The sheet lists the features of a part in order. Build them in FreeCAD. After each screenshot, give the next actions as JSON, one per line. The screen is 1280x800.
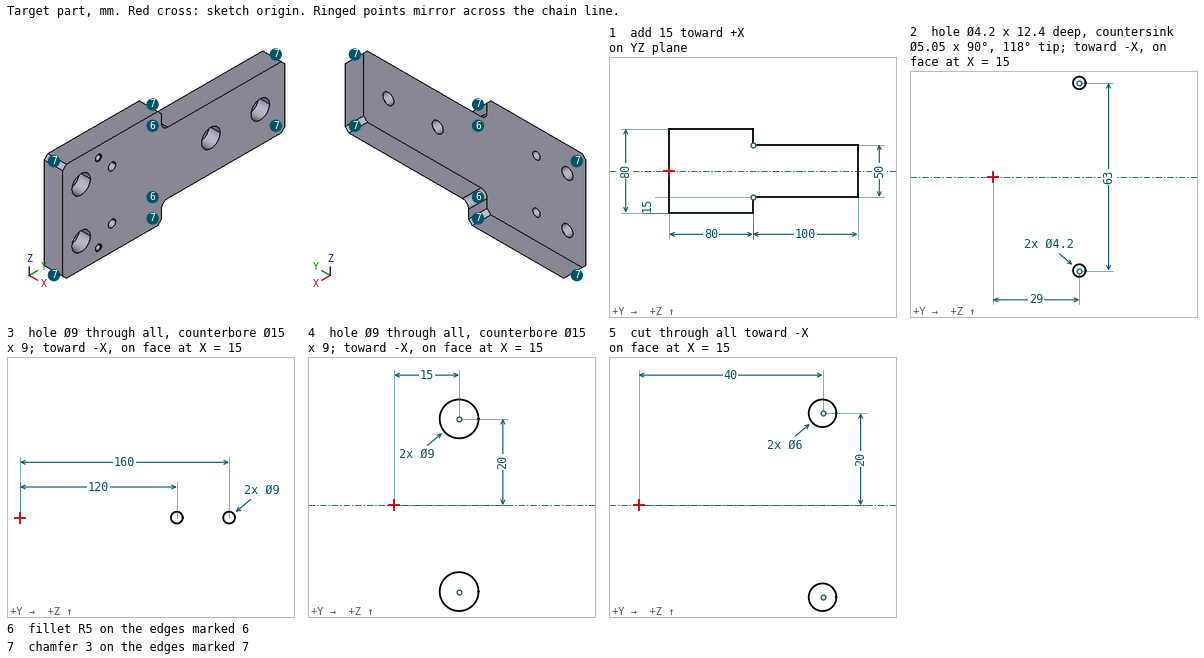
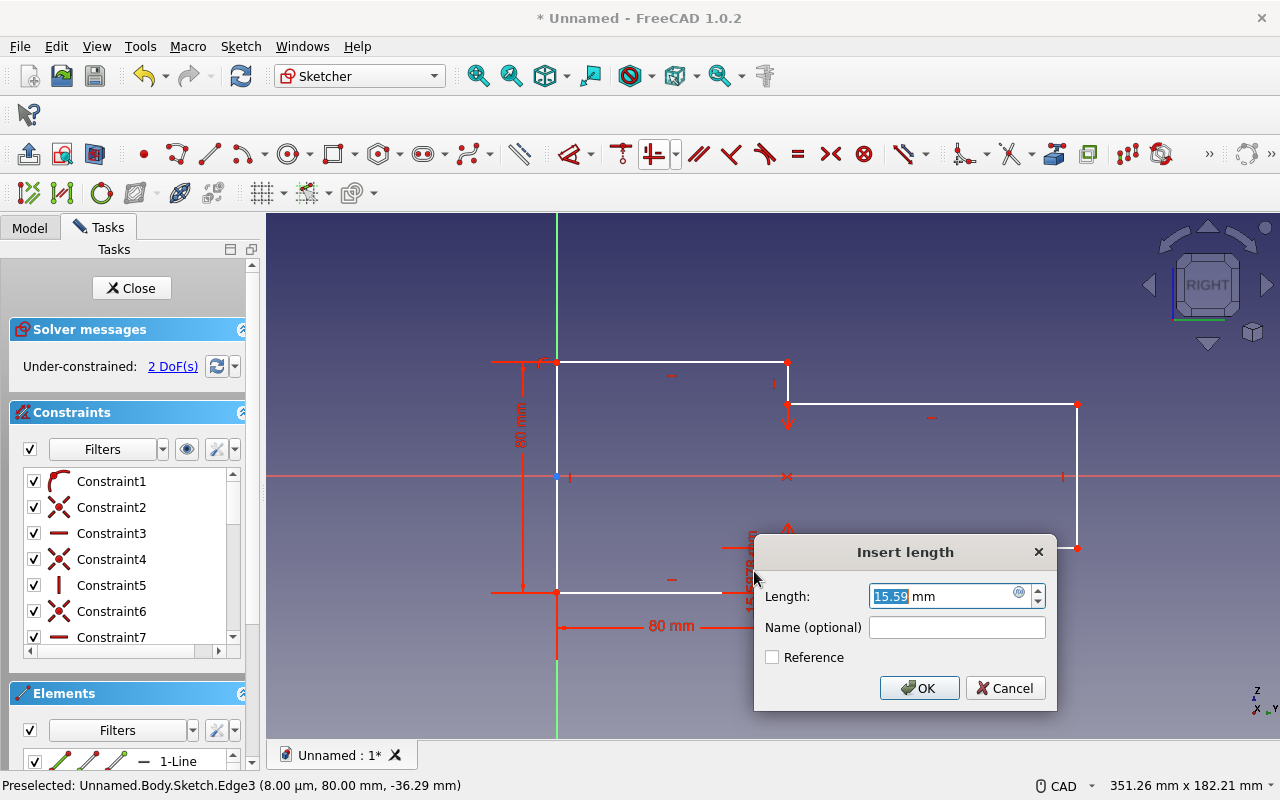
{"action": "type", "text": "15"}
{"action": "key", "text": "Return"}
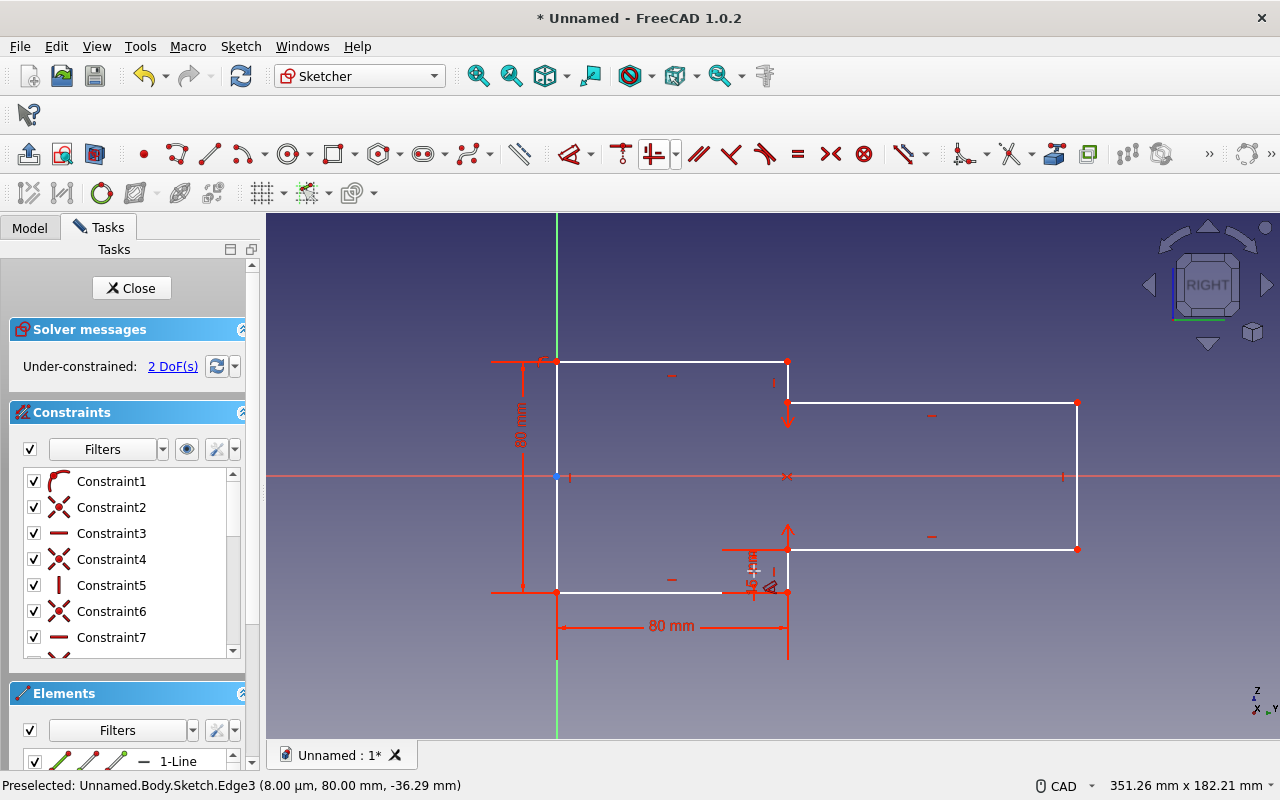
{"action": "left_click", "coordinate": [1077, 506]}
{"action": "left_click", "coordinate": [1111, 442]}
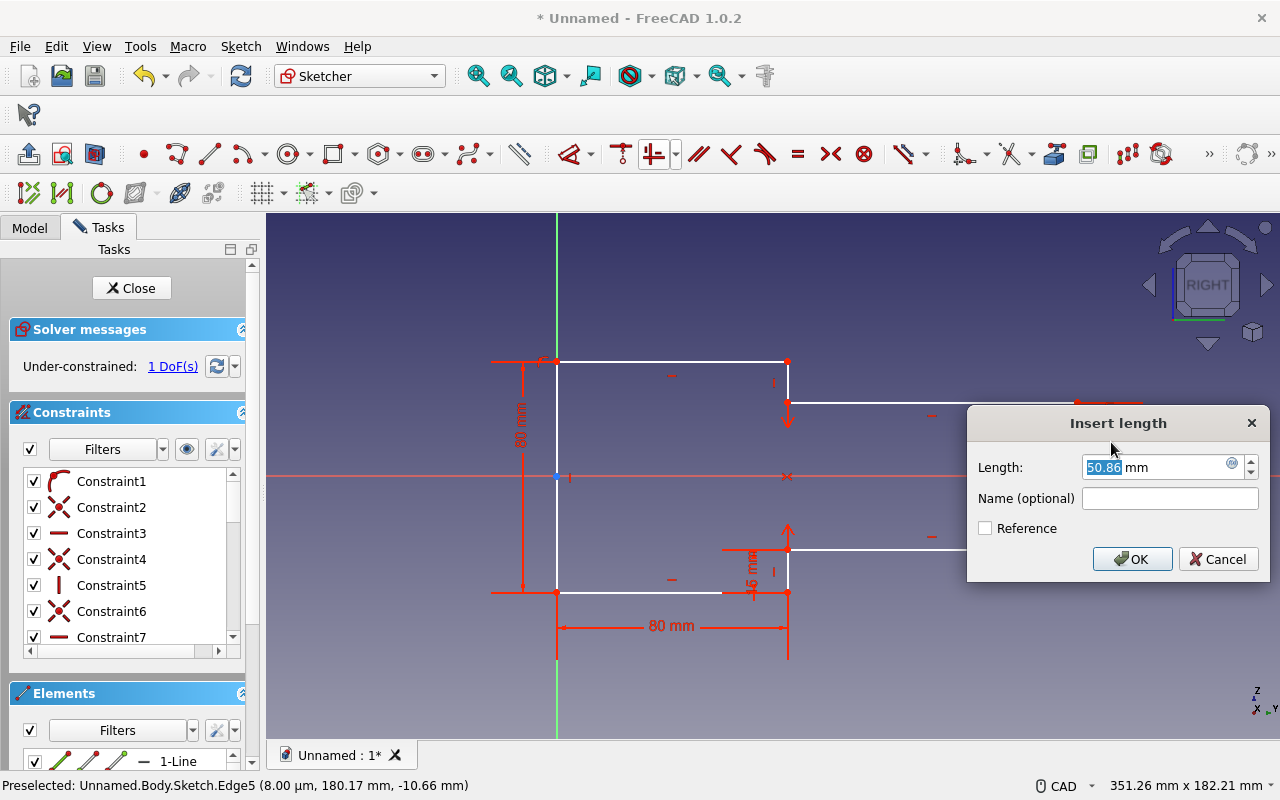
{"action": "type", "text": "50"}
{"action": "key", "text": "Return"}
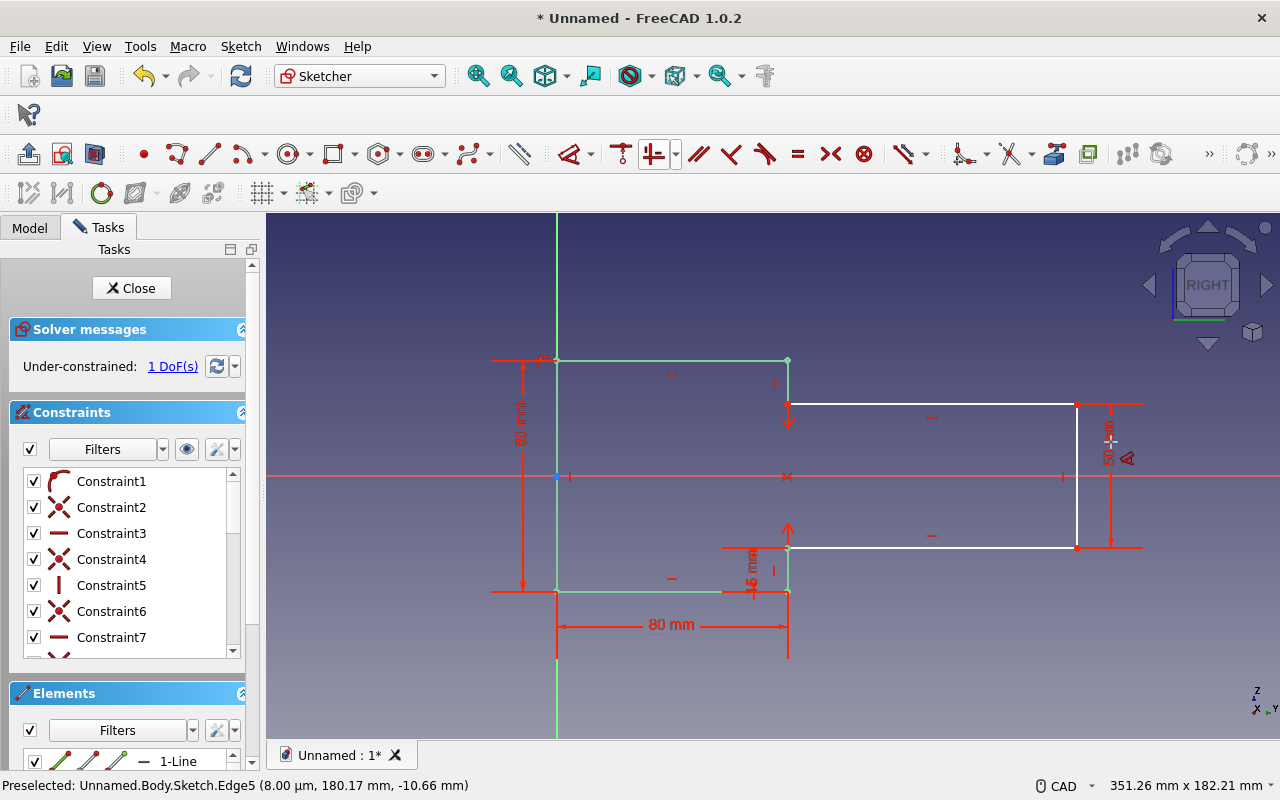
{"action": "left_click", "coordinate": [875, 548]}
{"action": "left_click", "coordinate": [932, 582]}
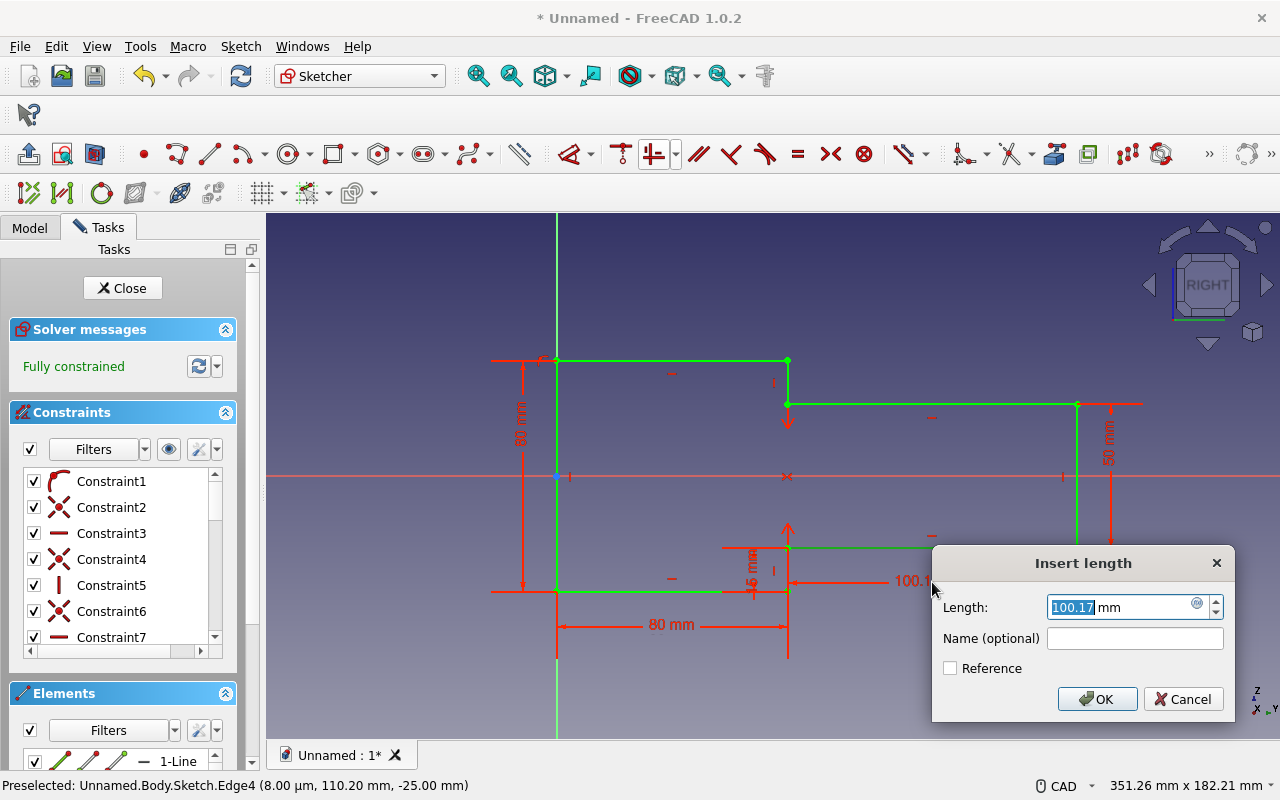
{"action": "type", "text": "100"}
{"action": "key", "text": "Return"}
{"action": "key", "text": "Escape"}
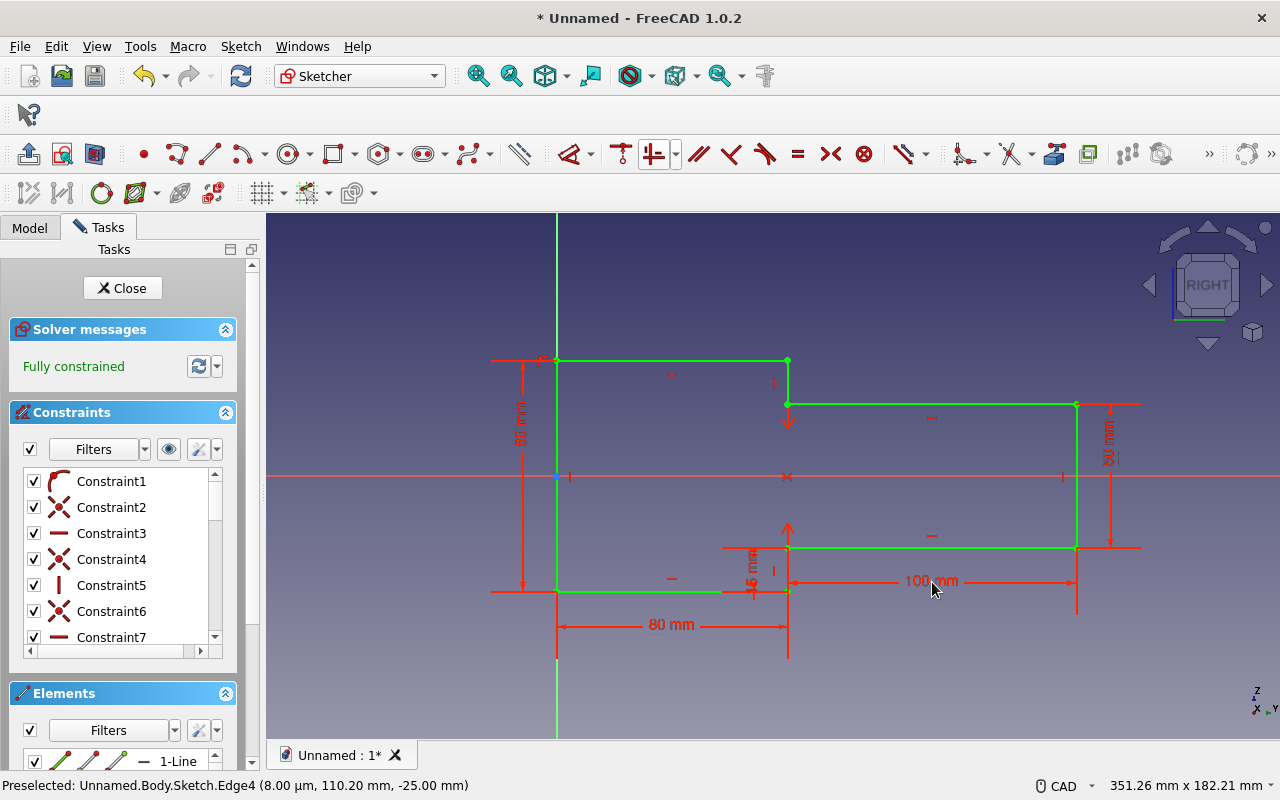
{"action": "left_click", "coordinate": [123, 288]}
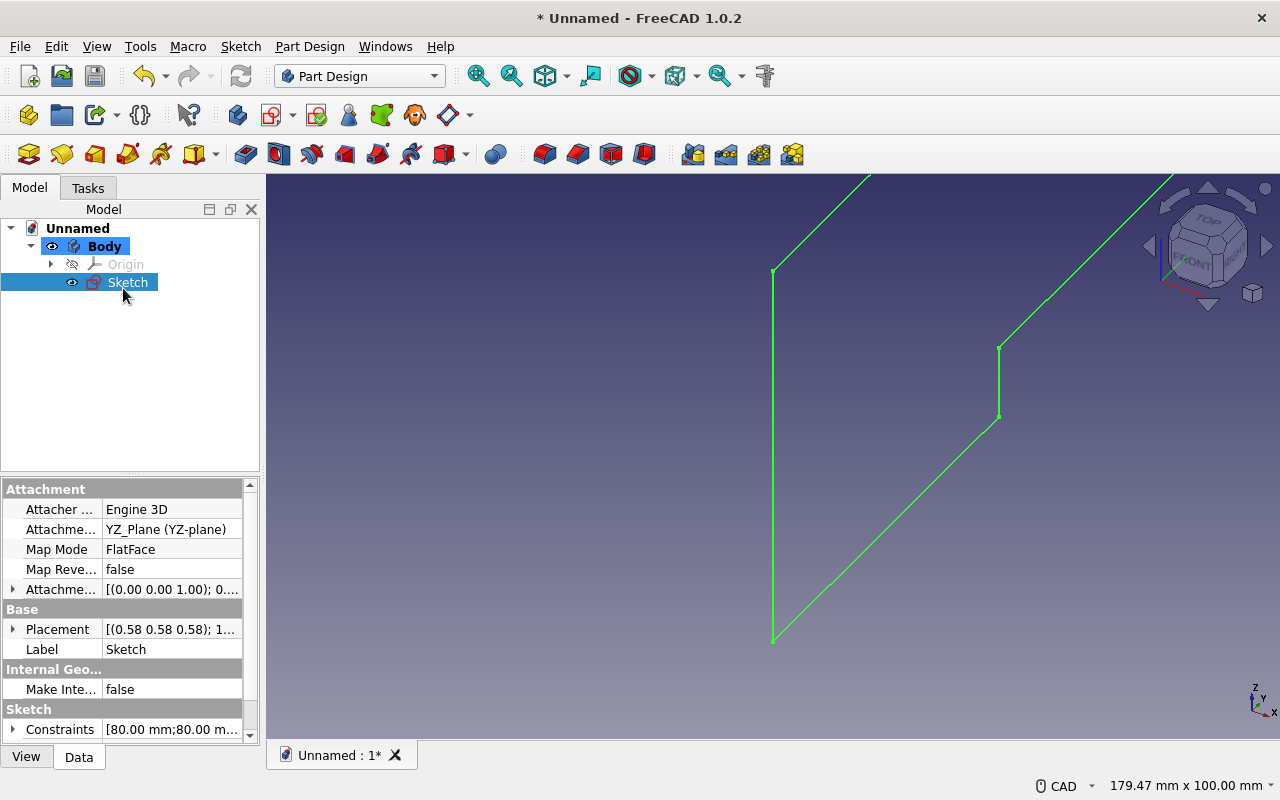
{"action": "left_click", "coordinate": [29, 154]}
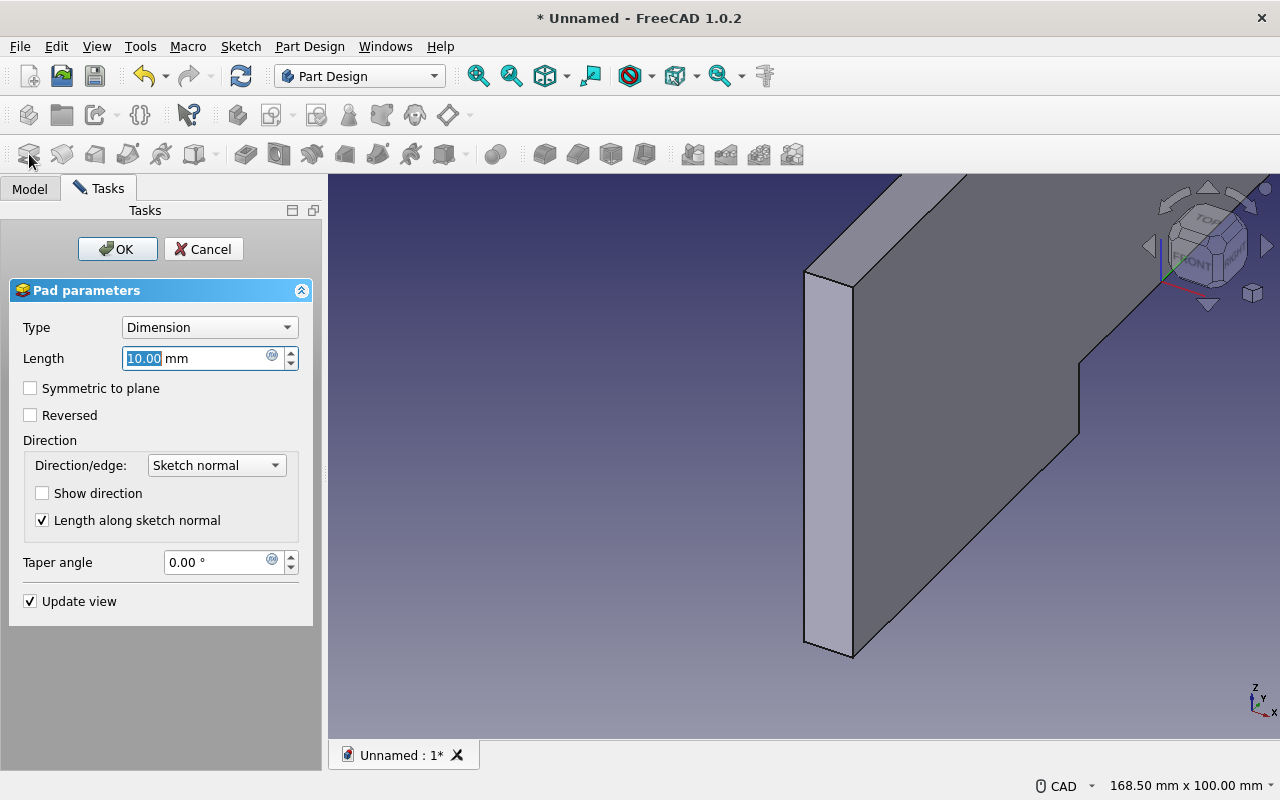
{"action": "type", "text": "15"}
{"action": "key", "text": "Tab"}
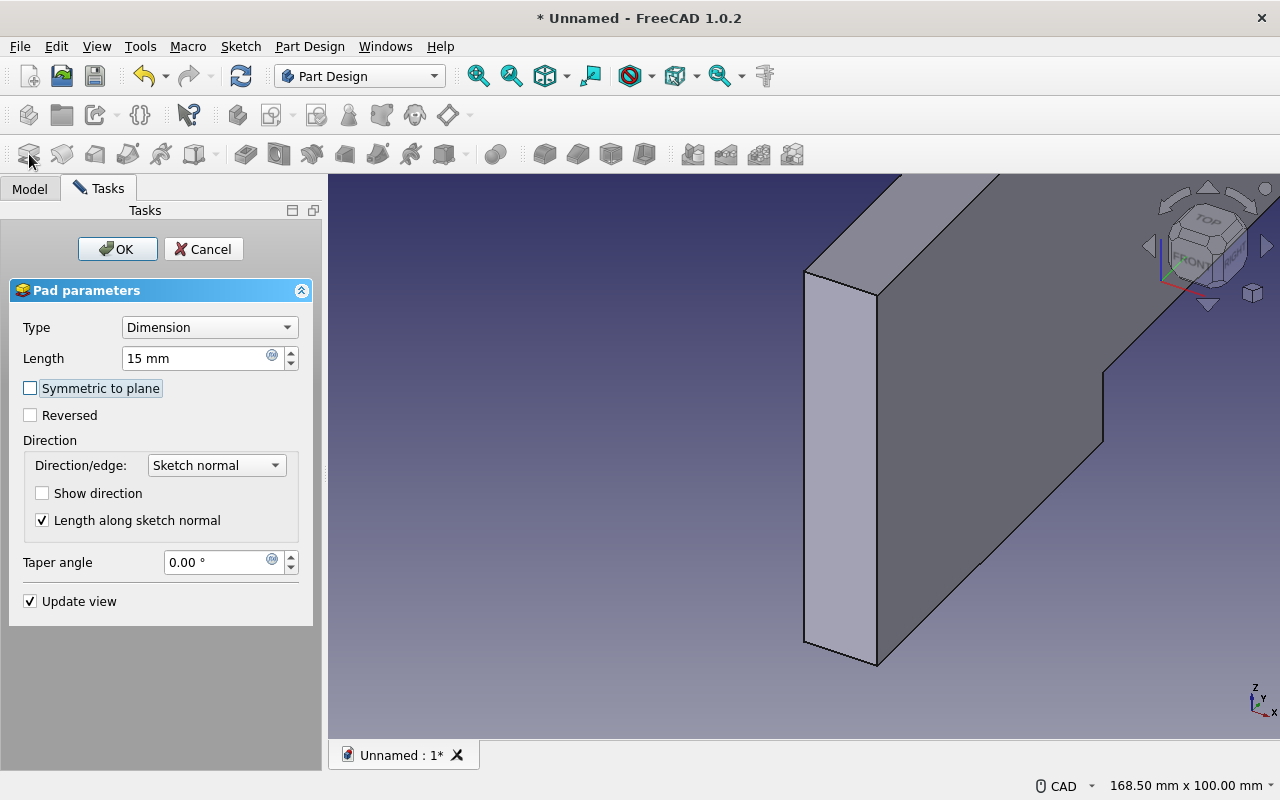
{"action": "left_click", "coordinate": [118, 249]}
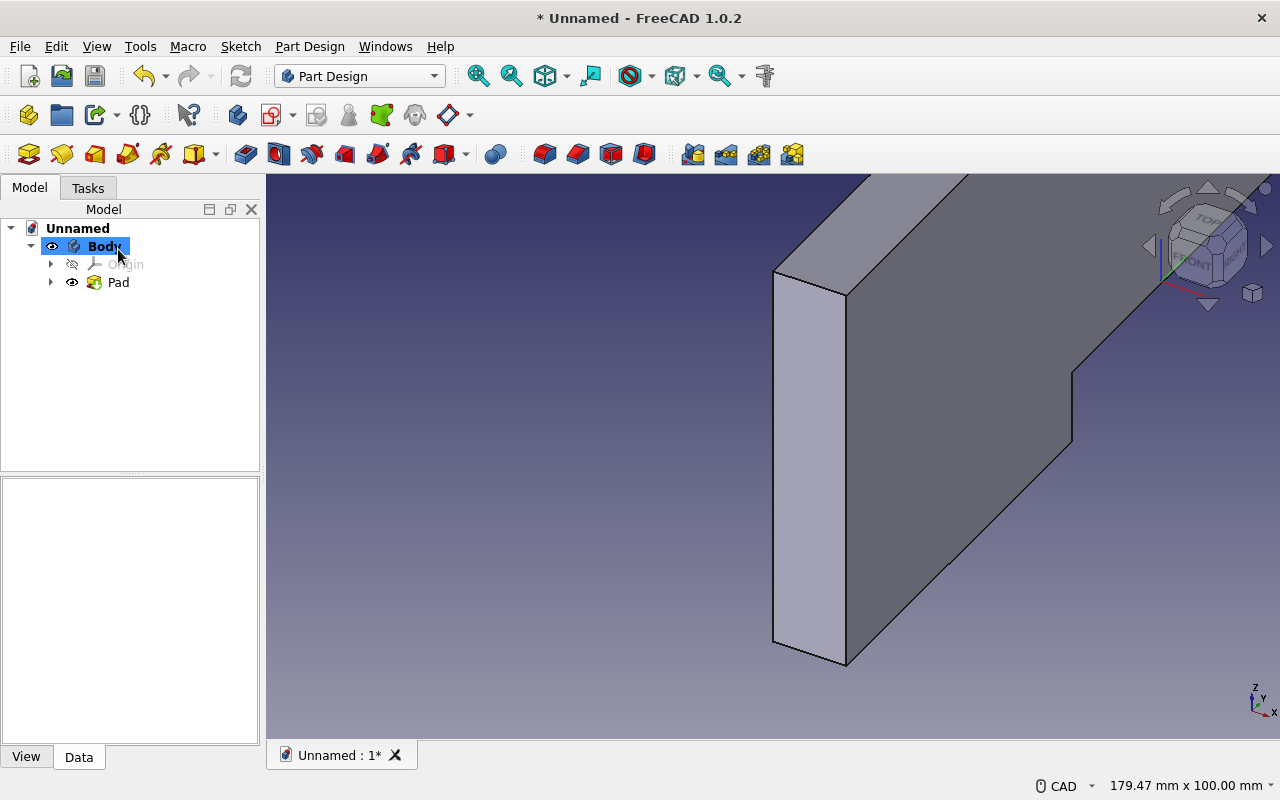
{"action": "left_click", "coordinate": [479, 76]}